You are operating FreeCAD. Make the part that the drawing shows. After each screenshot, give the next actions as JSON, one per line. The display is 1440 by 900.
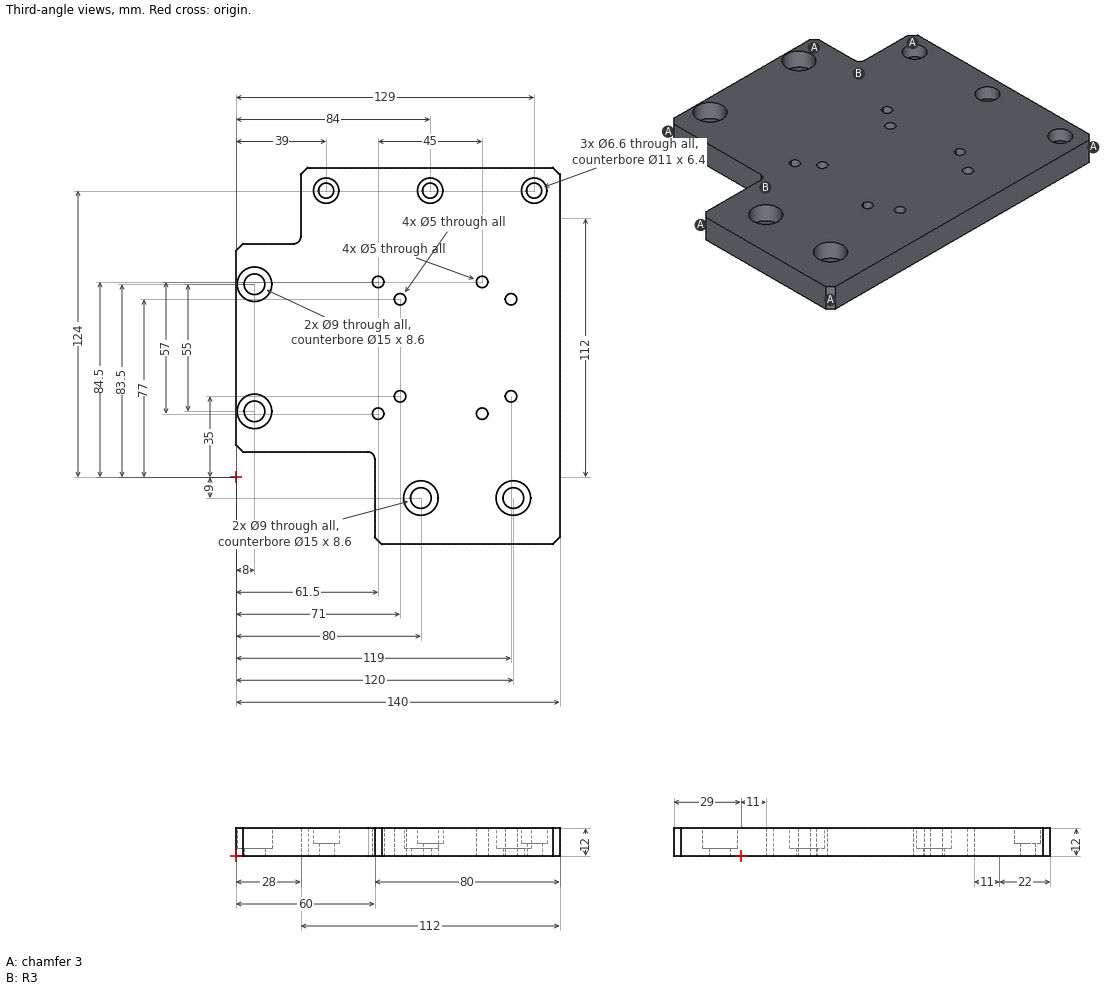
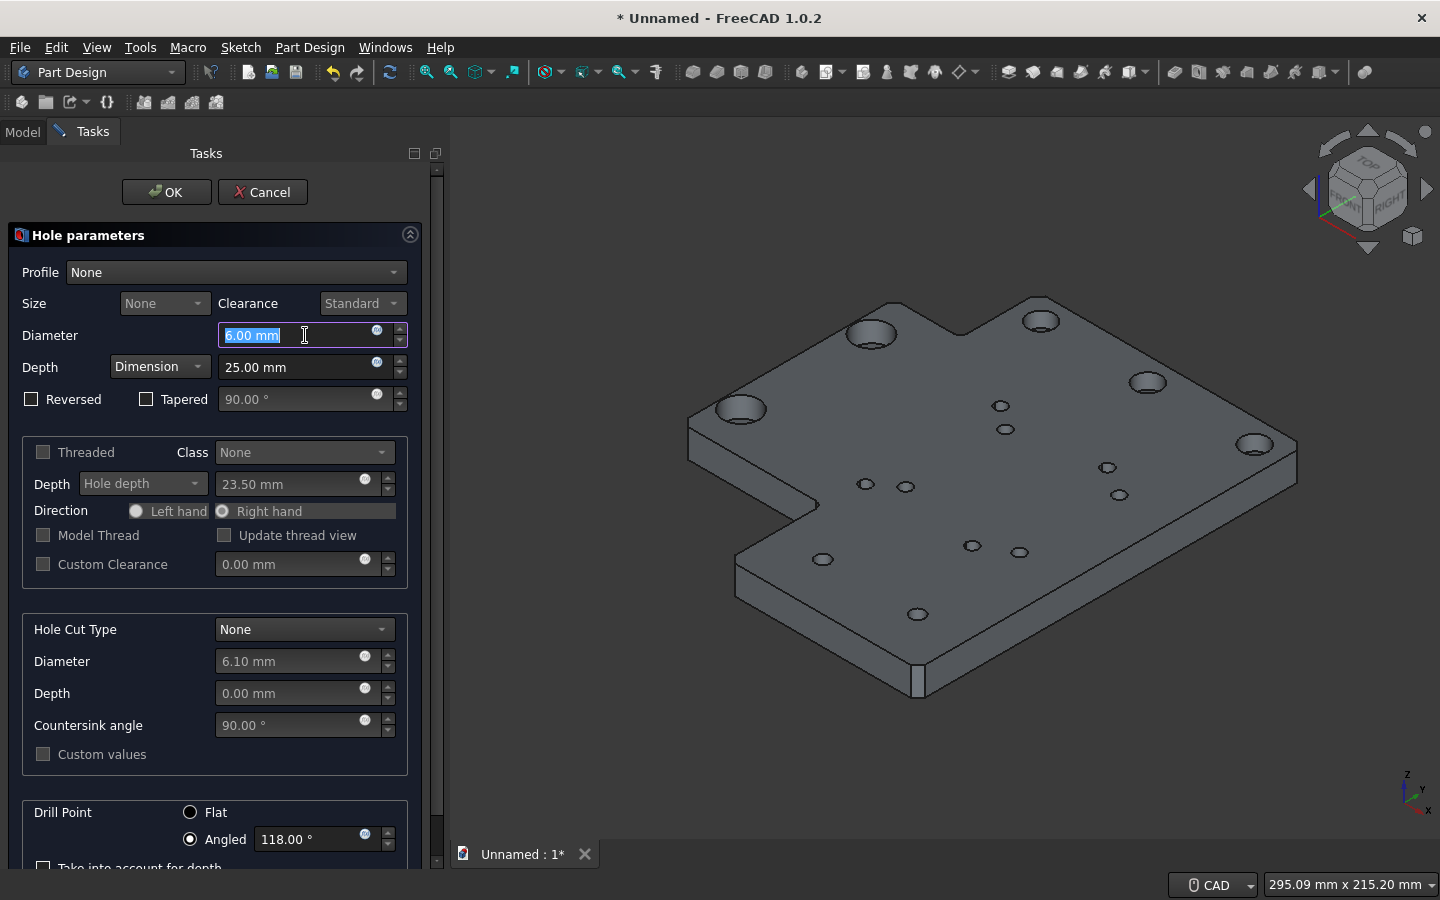
{"action": "type", "text": "9"}
{"action": "key", "text": "Tab"}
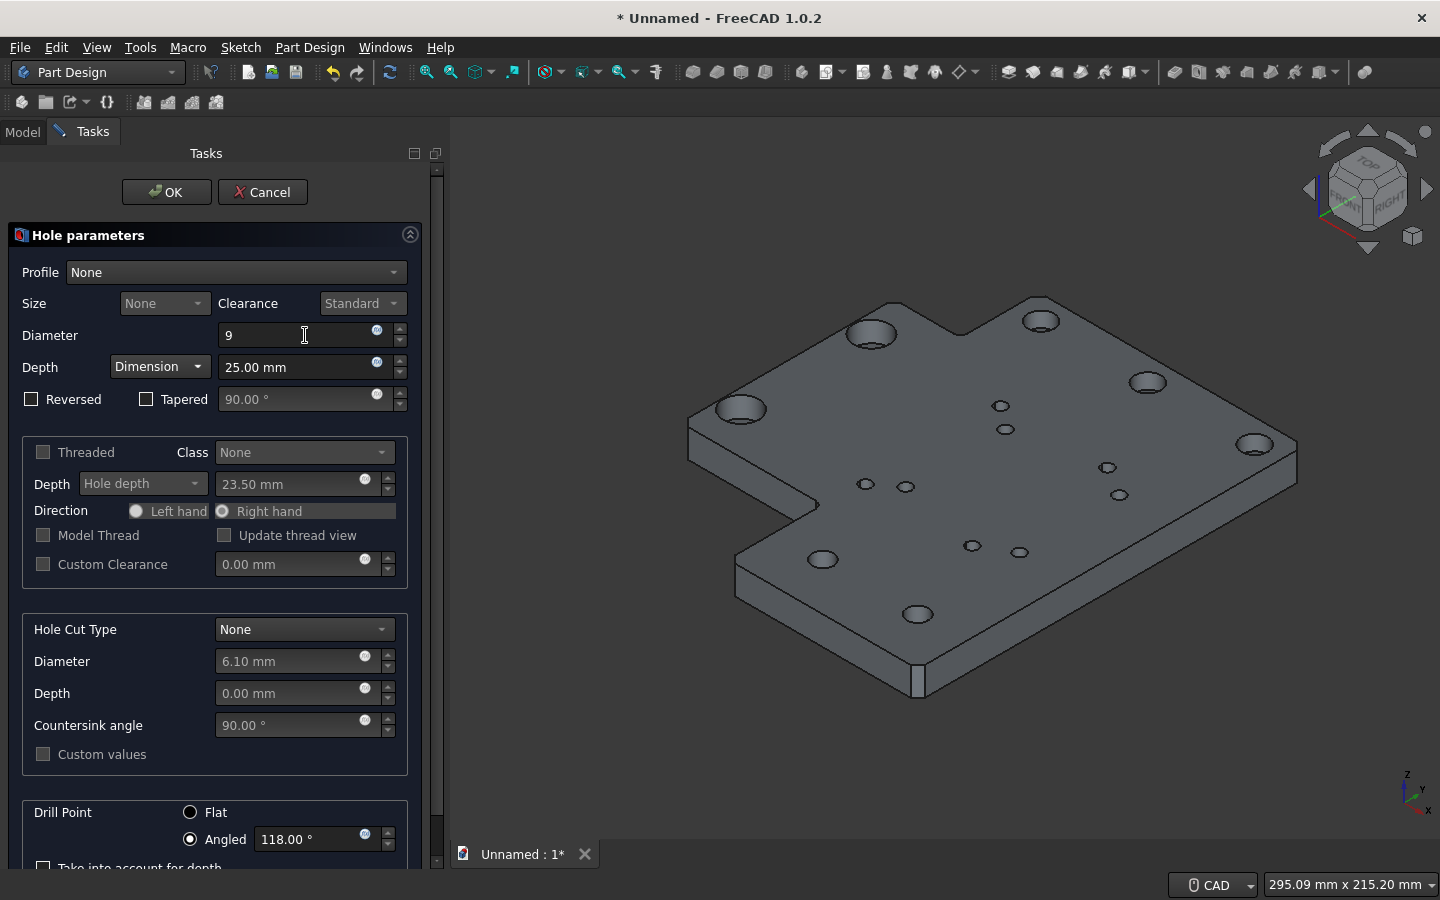
{"action": "left_click", "coordinate": [161, 366]}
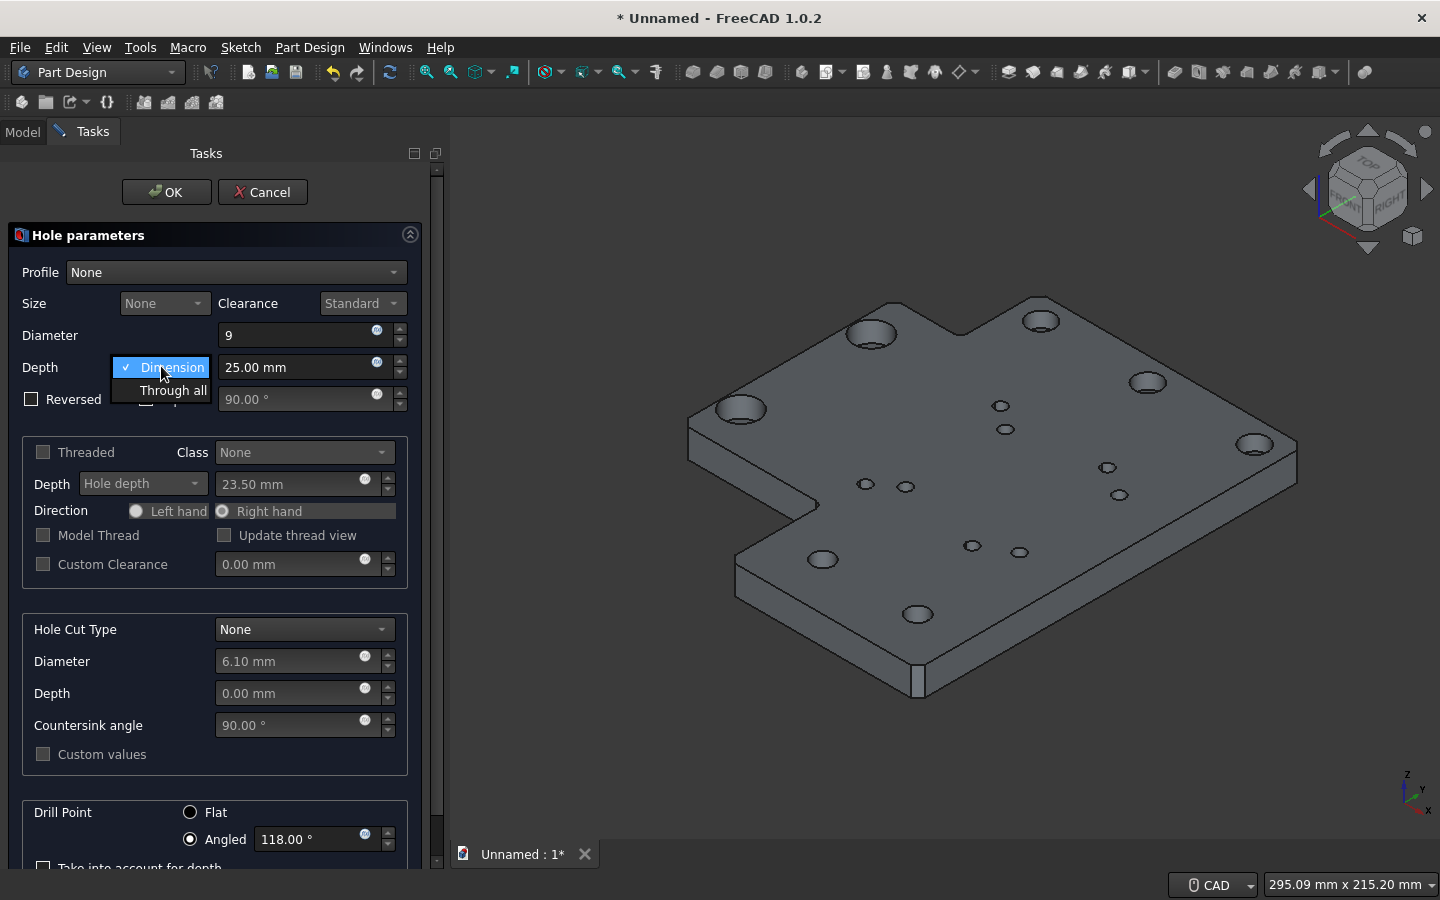
{"action": "left_click", "coordinate": [160, 390]}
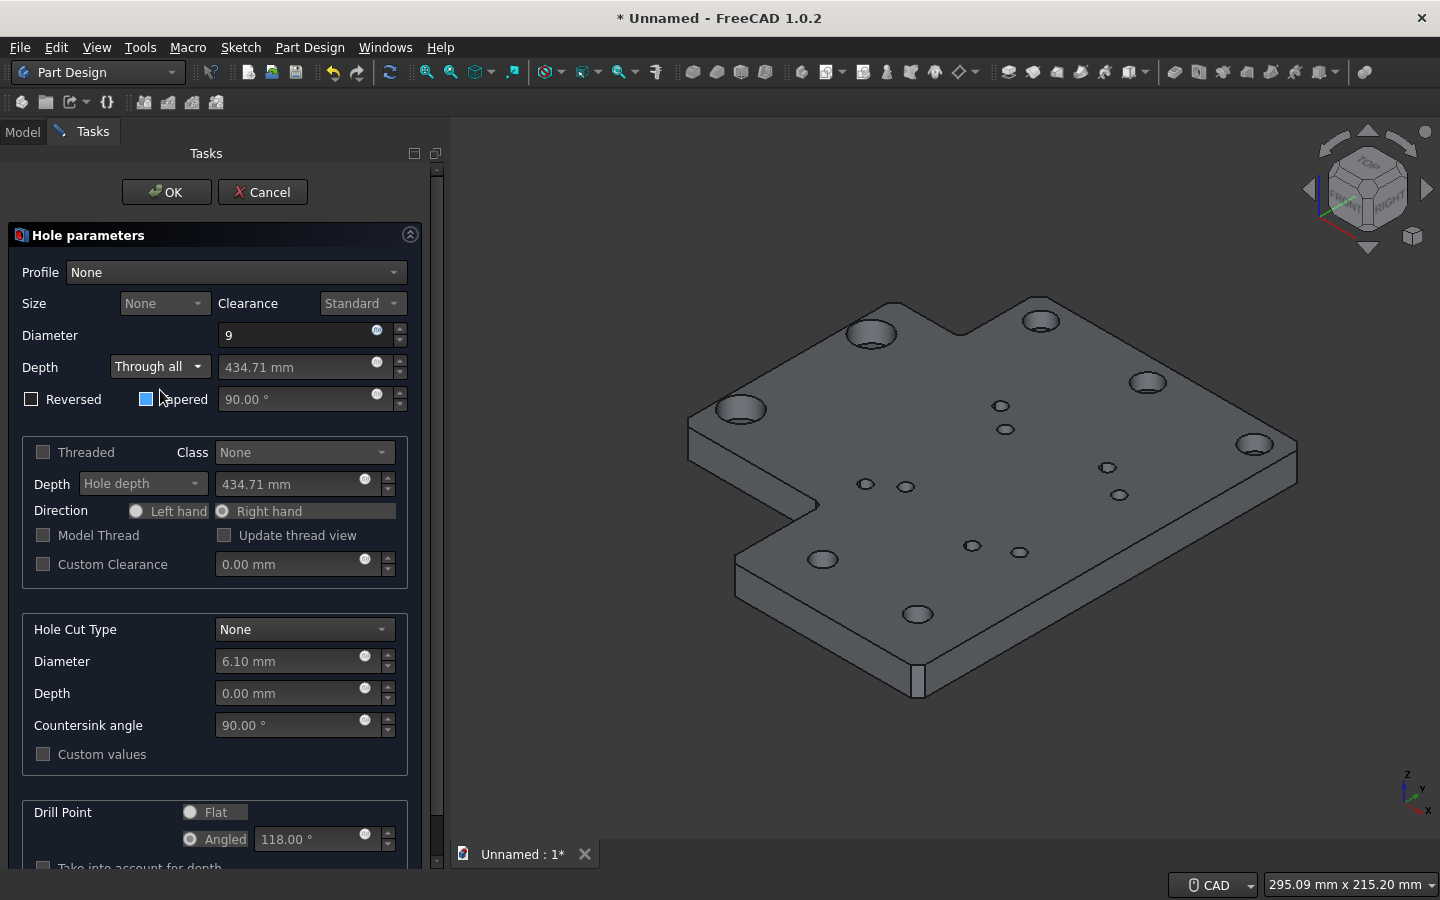
{"action": "left_click", "coordinate": [306, 630]}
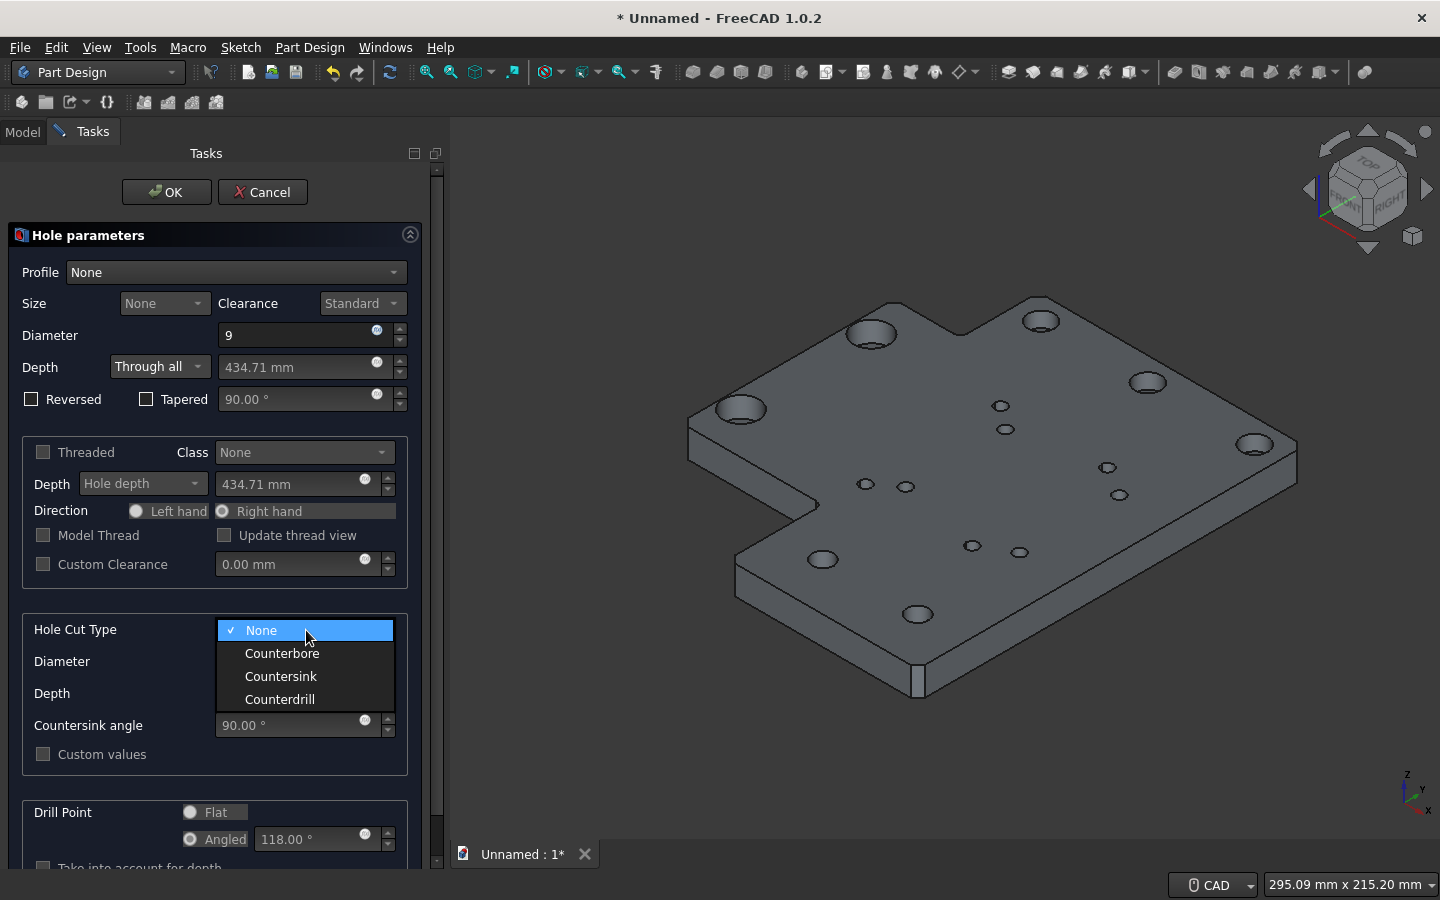
{"action": "left_click", "coordinate": [304, 654]}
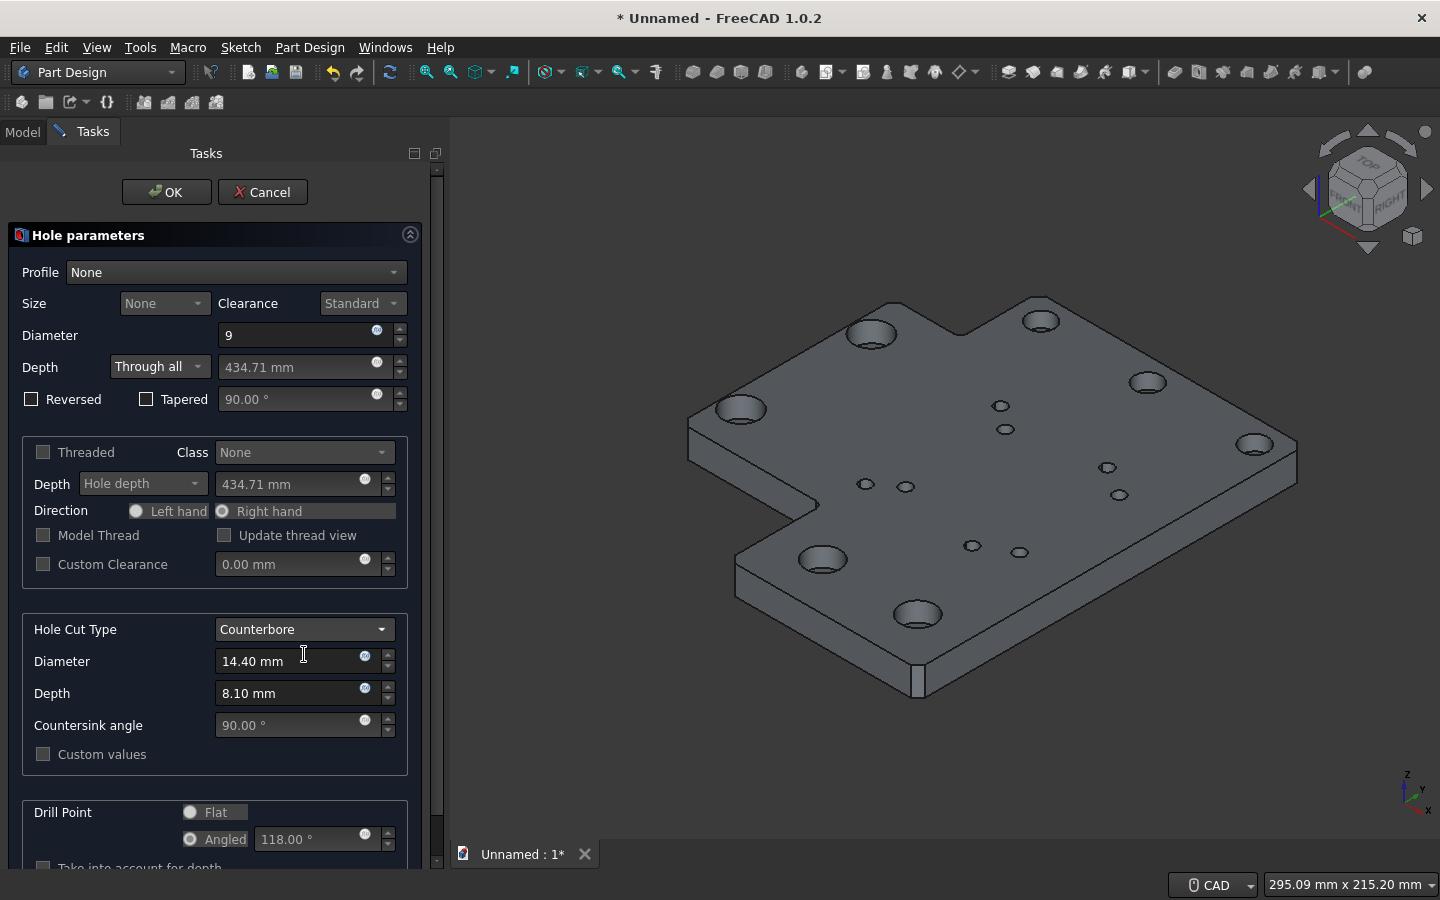
{"action": "triple_click", "coordinate": [298, 661]}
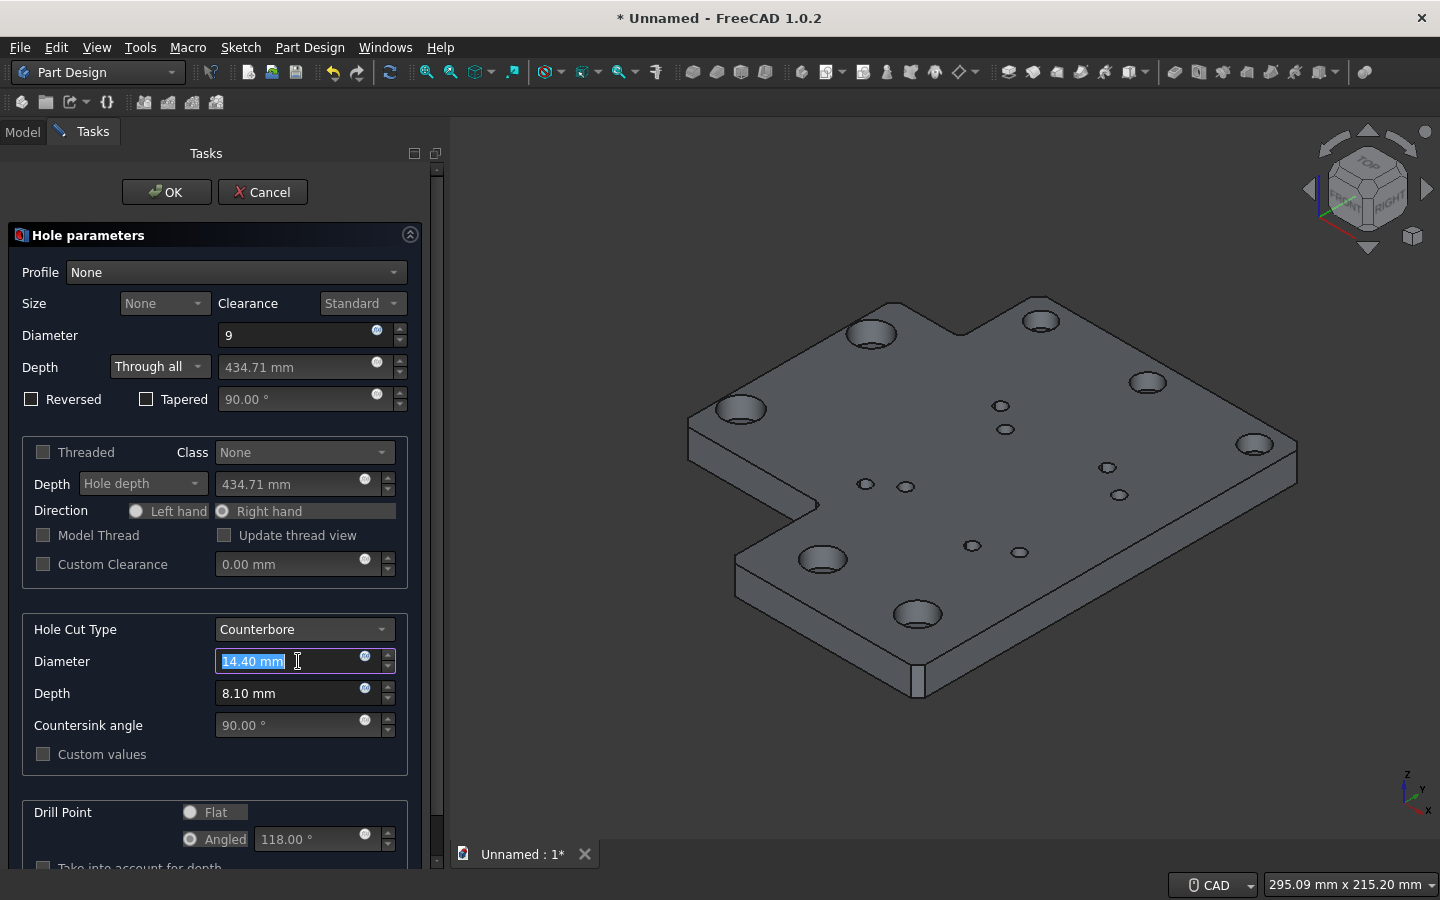
{"action": "type", "text": "15"}
{"action": "key", "text": "Tab"}